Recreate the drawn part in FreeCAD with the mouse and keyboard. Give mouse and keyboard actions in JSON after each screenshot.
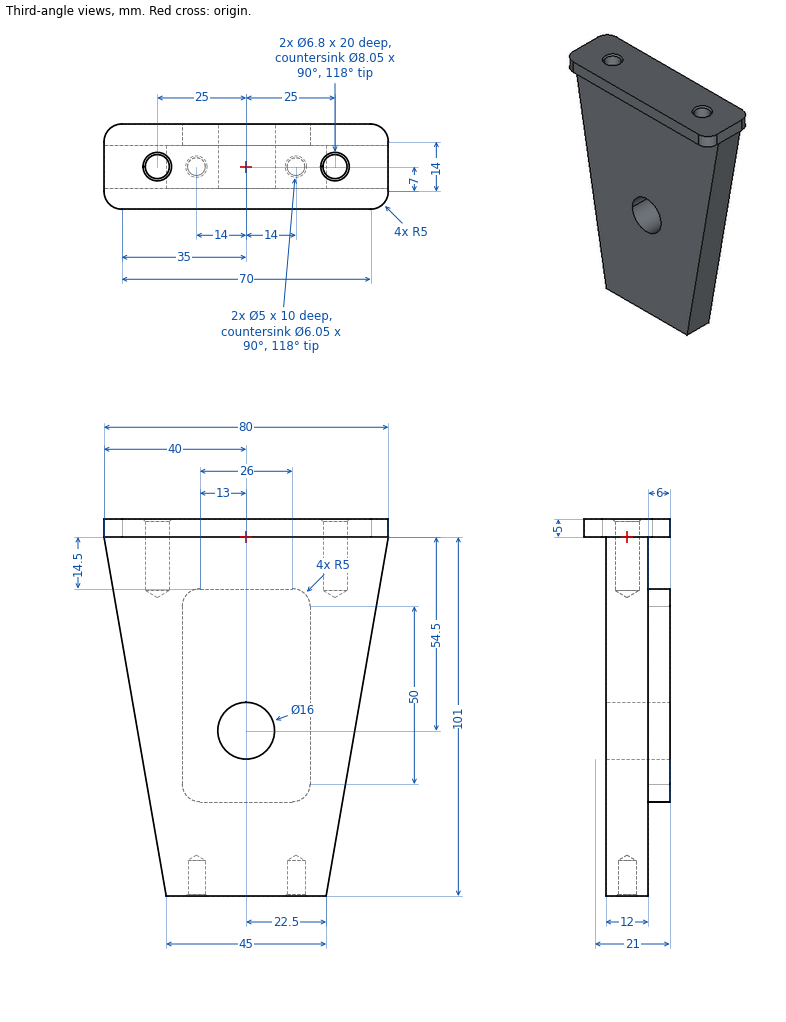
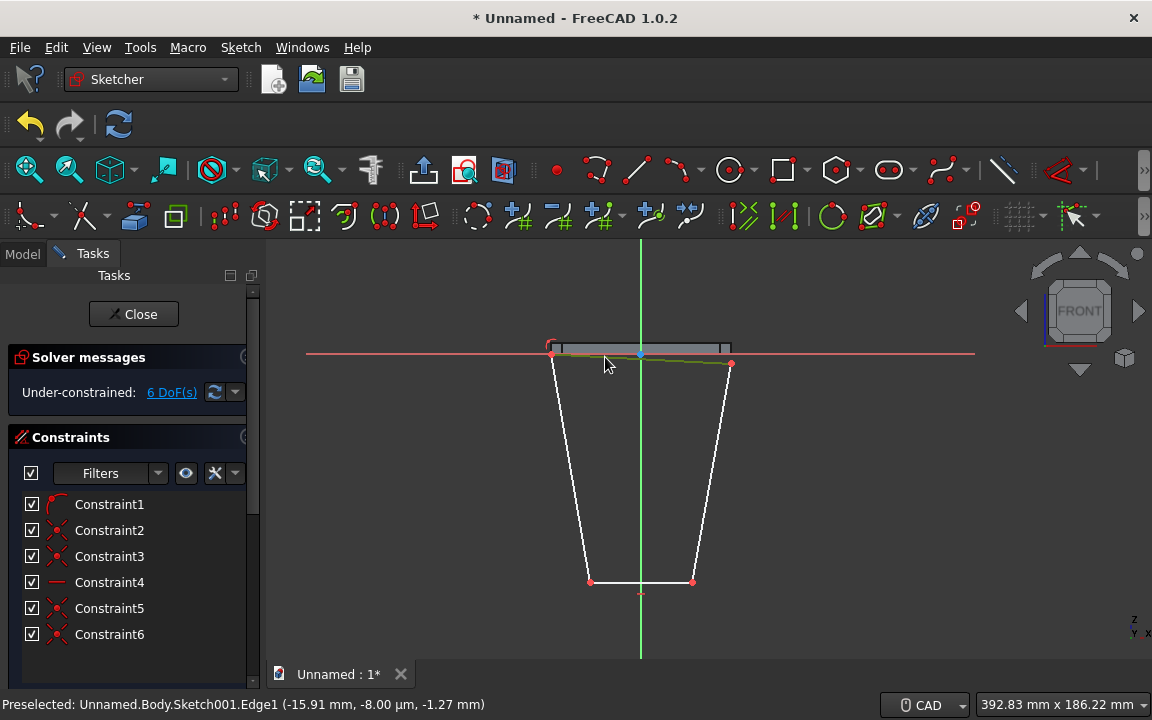
{"action": "key", "text": "h"}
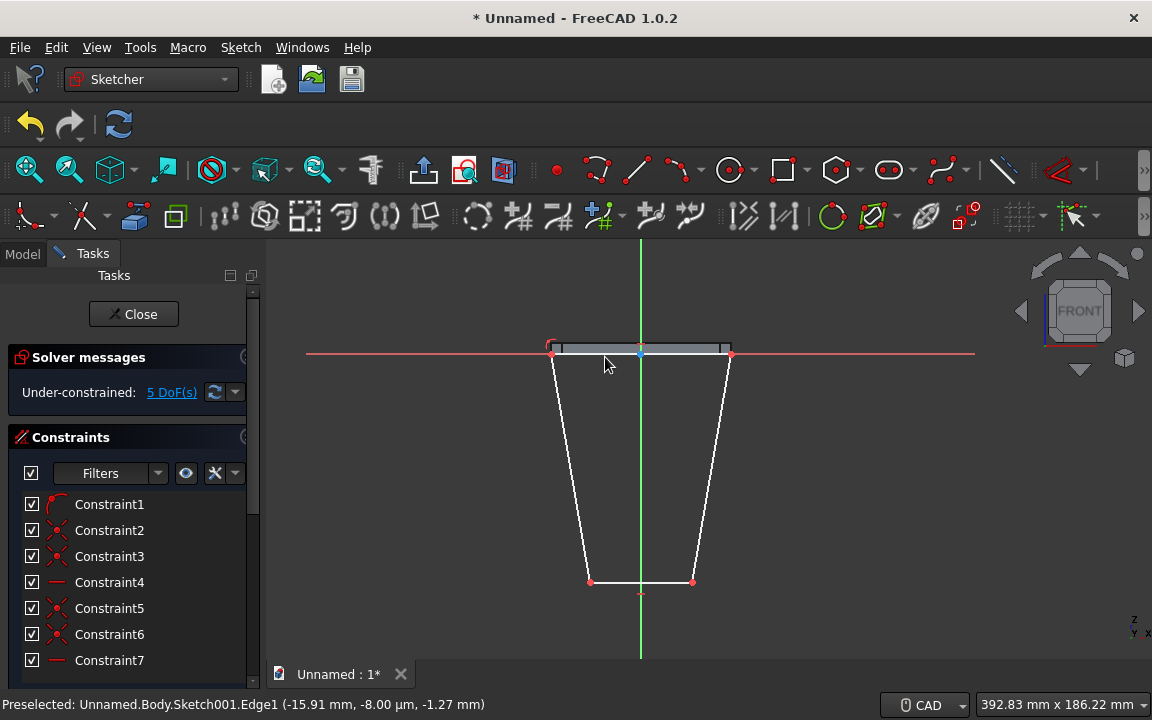
{"action": "left_click", "coordinate": [1058, 170]}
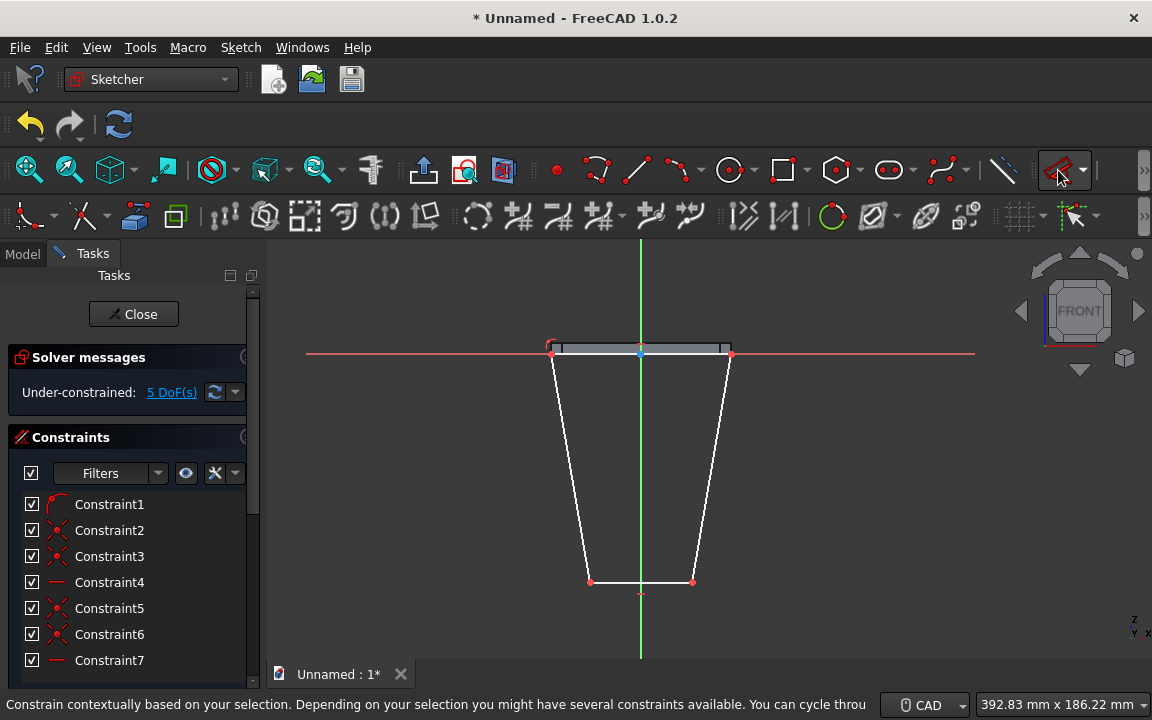
{"action": "left_click", "coordinate": [605, 354]}
{"action": "left_click", "coordinate": [600, 320]}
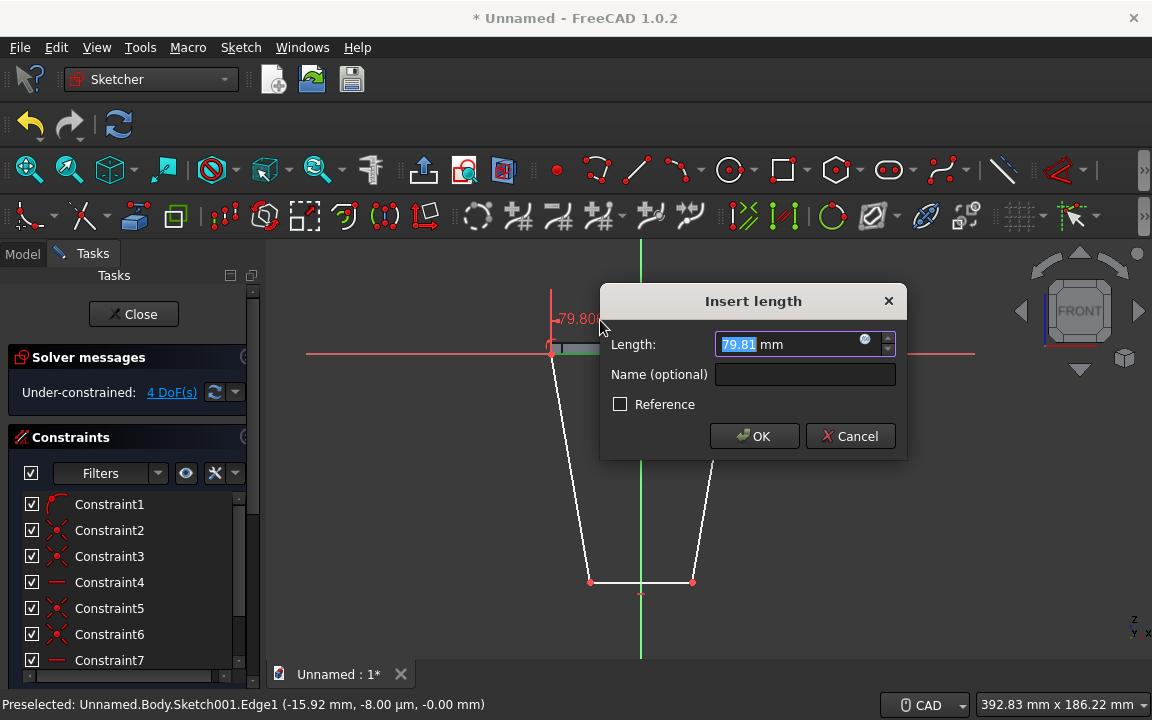
{"action": "type", "text": "80"}
{"action": "key", "text": "Return"}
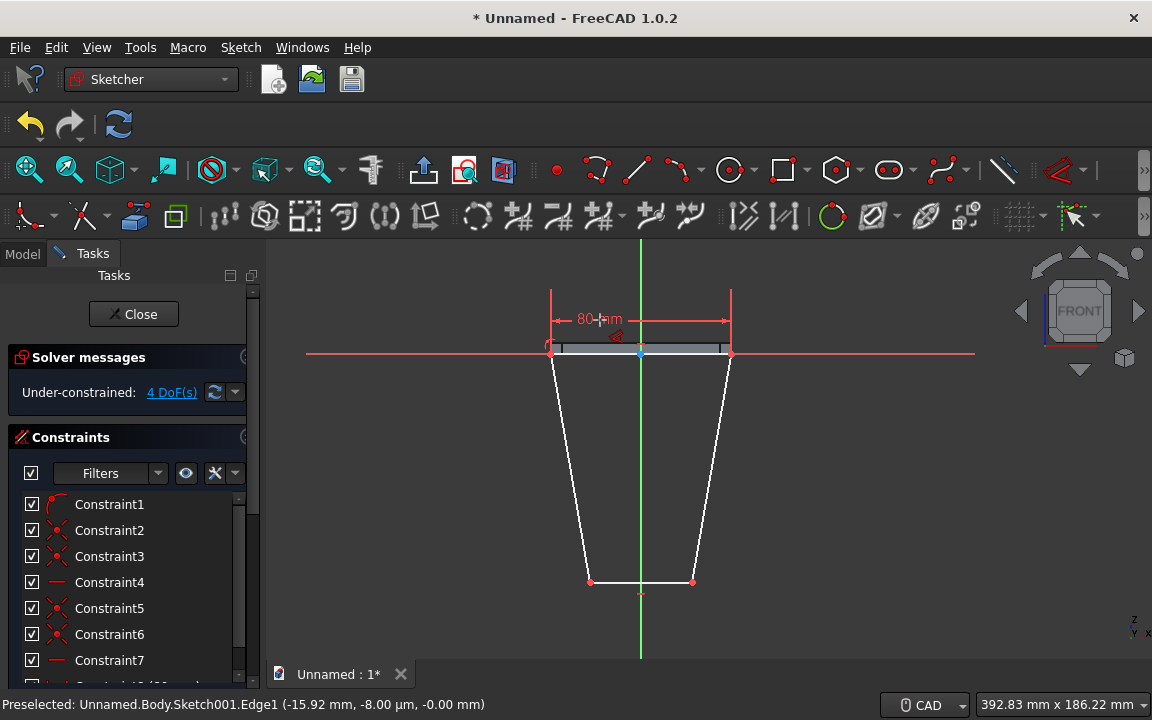
{"action": "left_click", "coordinate": [661, 583]}
{"action": "left_click", "coordinate": [618, 617]}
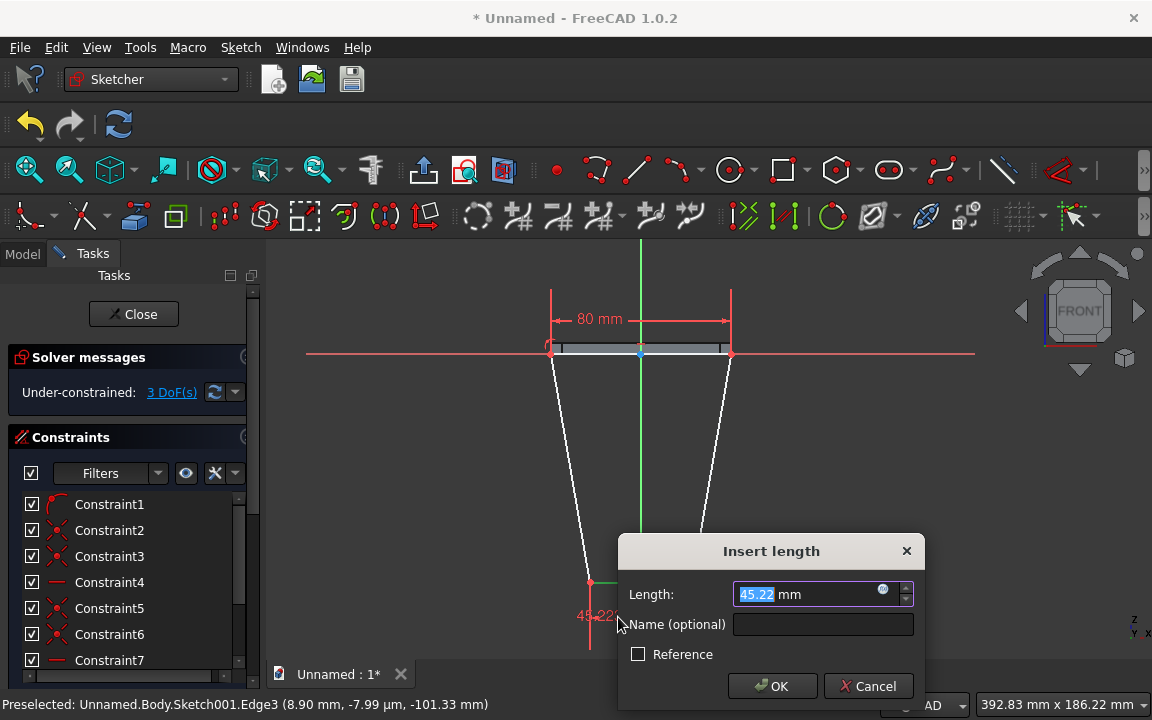
{"action": "type", "text": "45"}
{"action": "key", "text": "Return"}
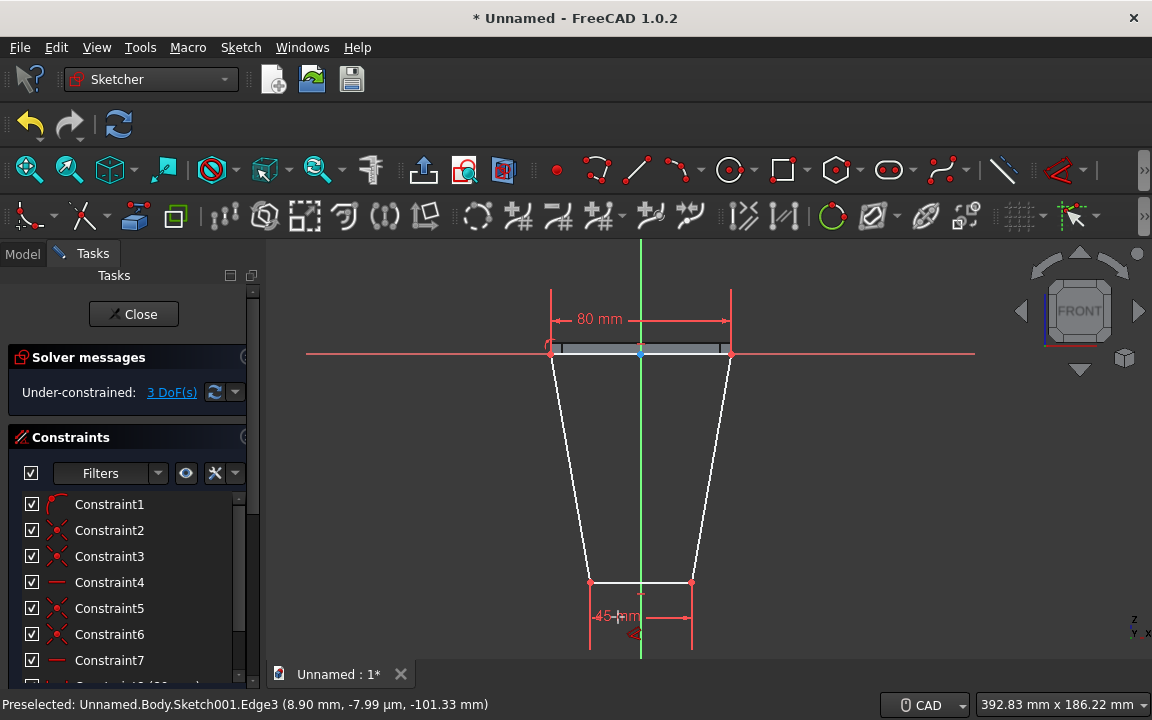
{"action": "left_click", "coordinate": [551, 354]}
{"action": "left_click", "coordinate": [596, 388]}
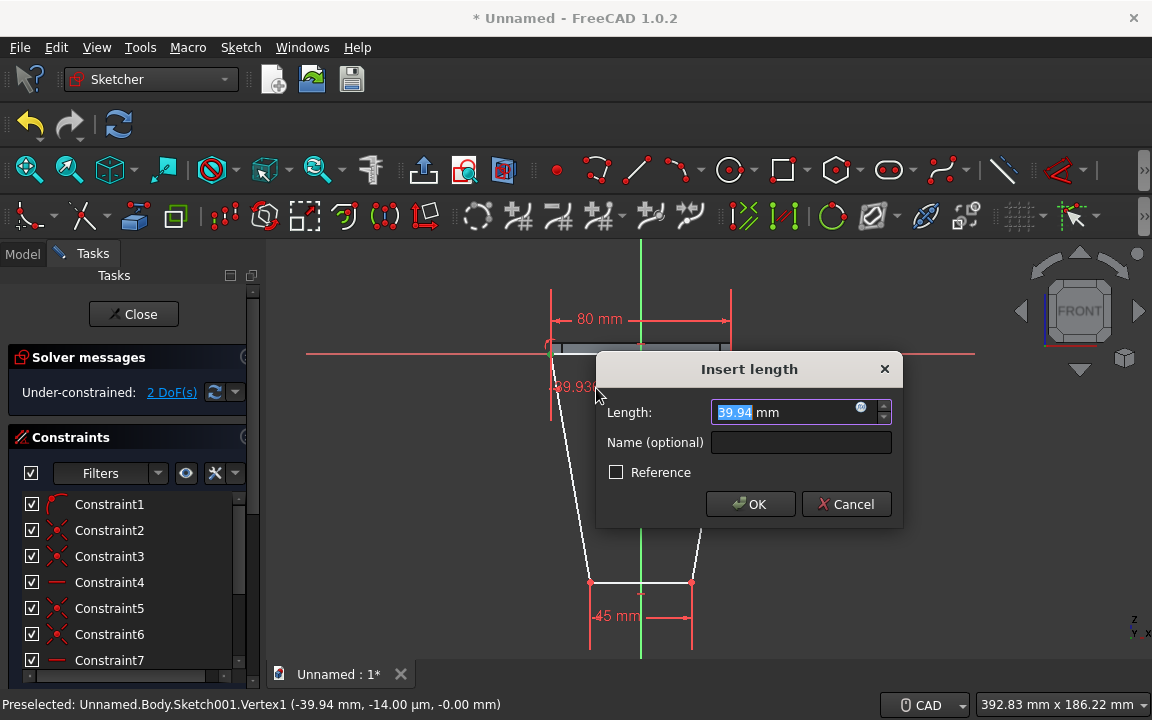
{"action": "type", "text": "40"}
{"action": "key", "text": "Return"}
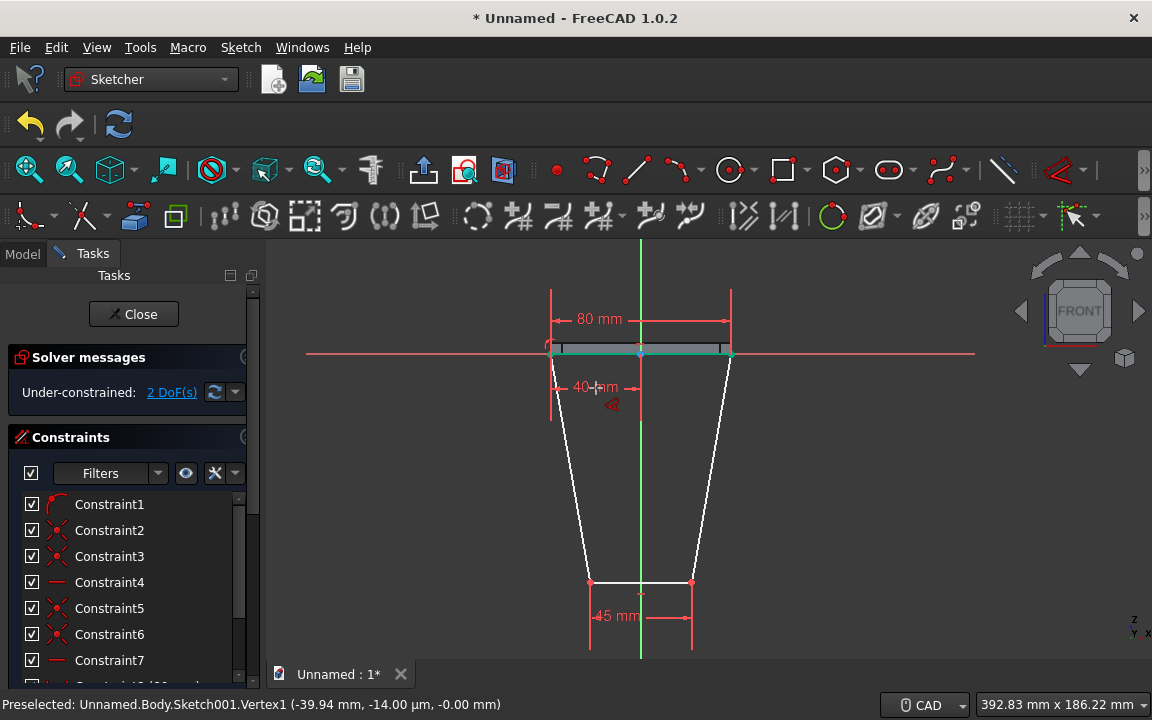
{"action": "left_click", "coordinate": [692, 583]}
{"action": "left_click", "coordinate": [726, 469]}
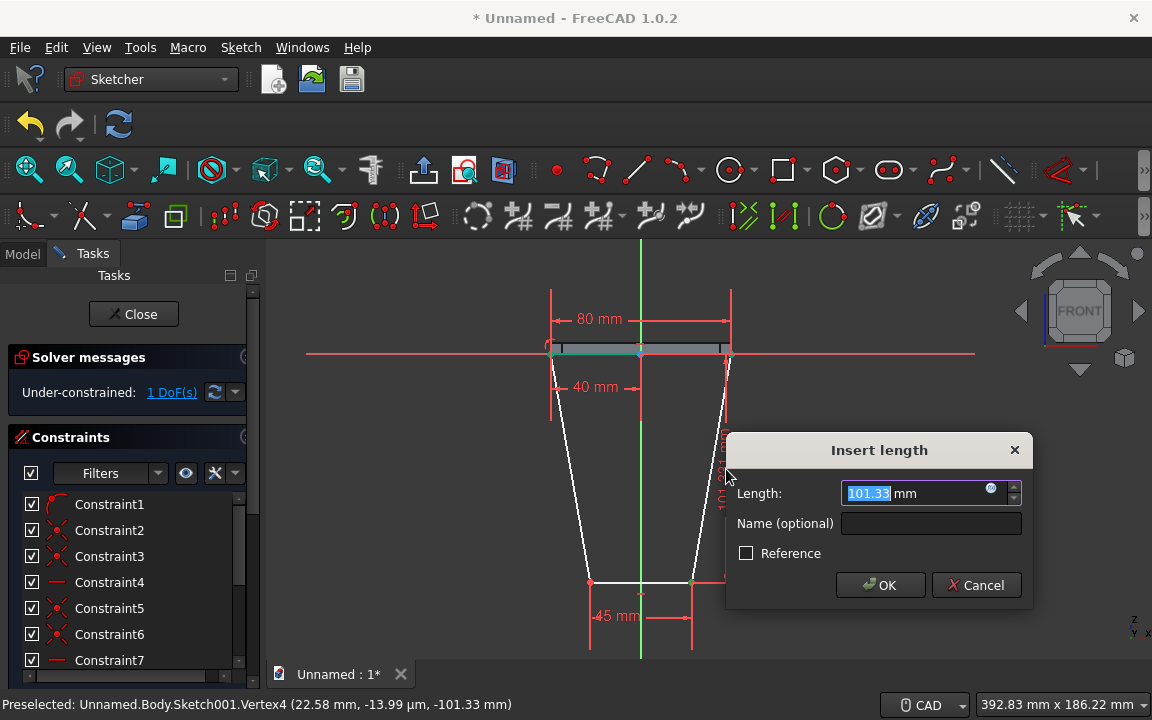
{"action": "type", "text": "101"}
{"action": "key", "text": "Return"}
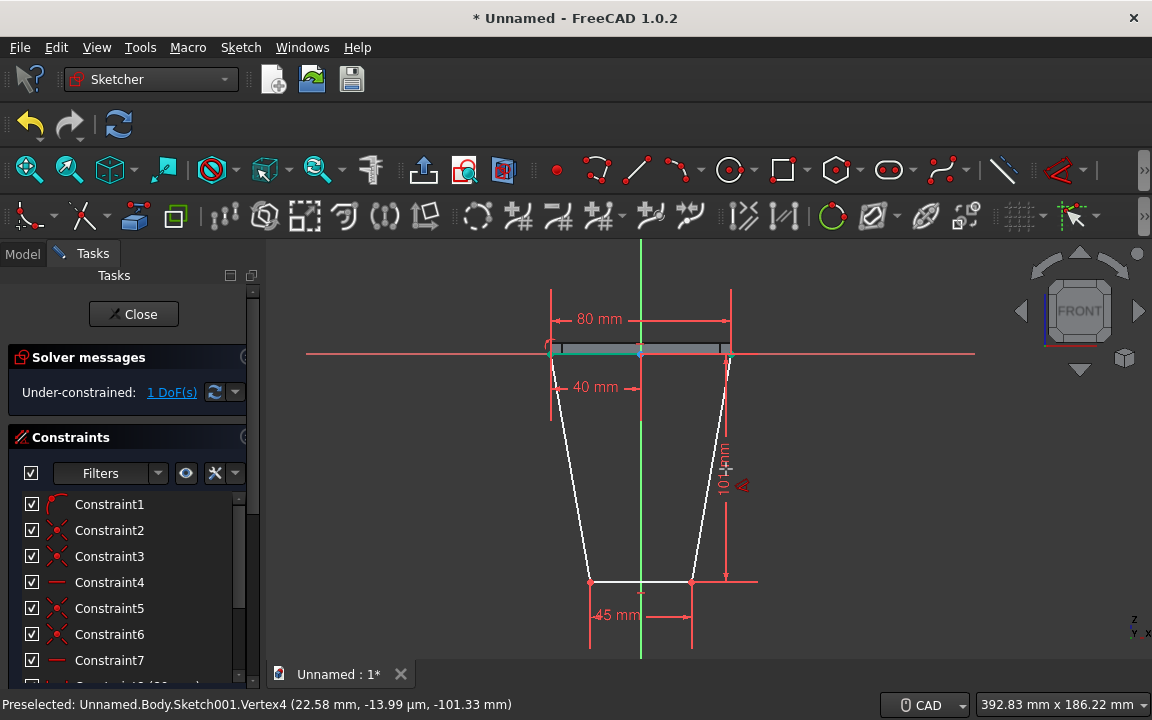
{"action": "left_click", "coordinate": [692, 582]}
{"action": "left_click", "coordinate": [678, 320]}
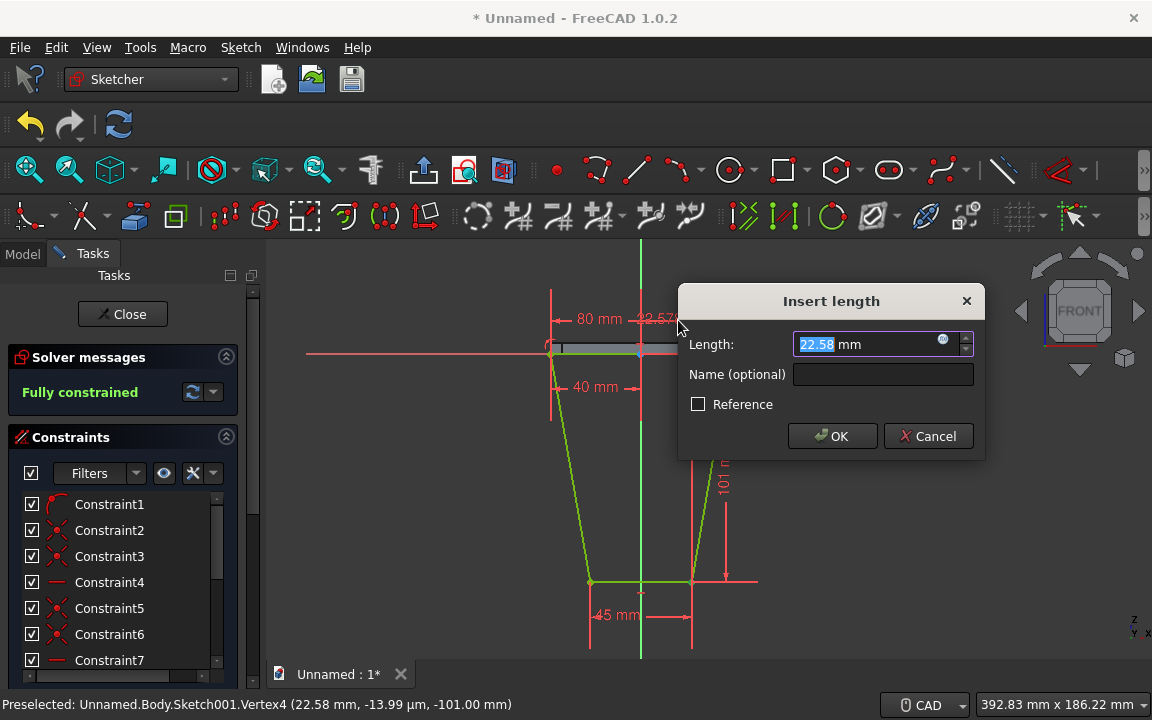
{"action": "type", "text": "22.5"}
{"action": "key", "text": "Return"}
{"action": "key", "text": "Escape"}